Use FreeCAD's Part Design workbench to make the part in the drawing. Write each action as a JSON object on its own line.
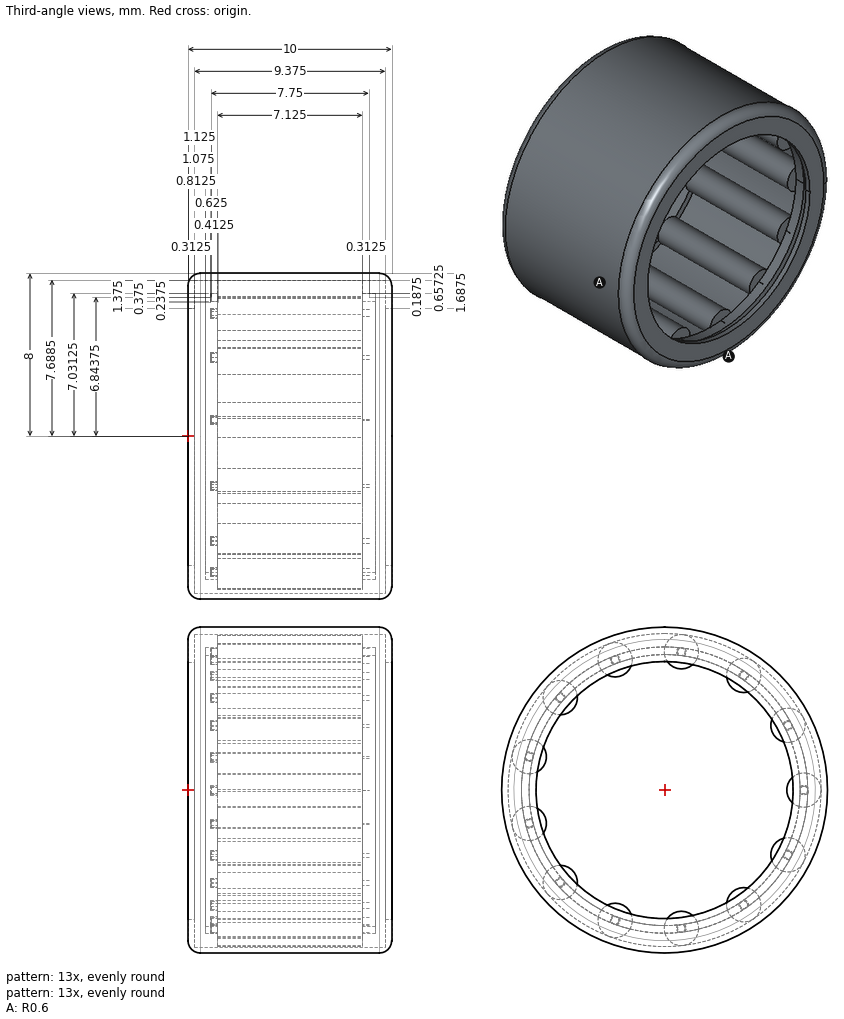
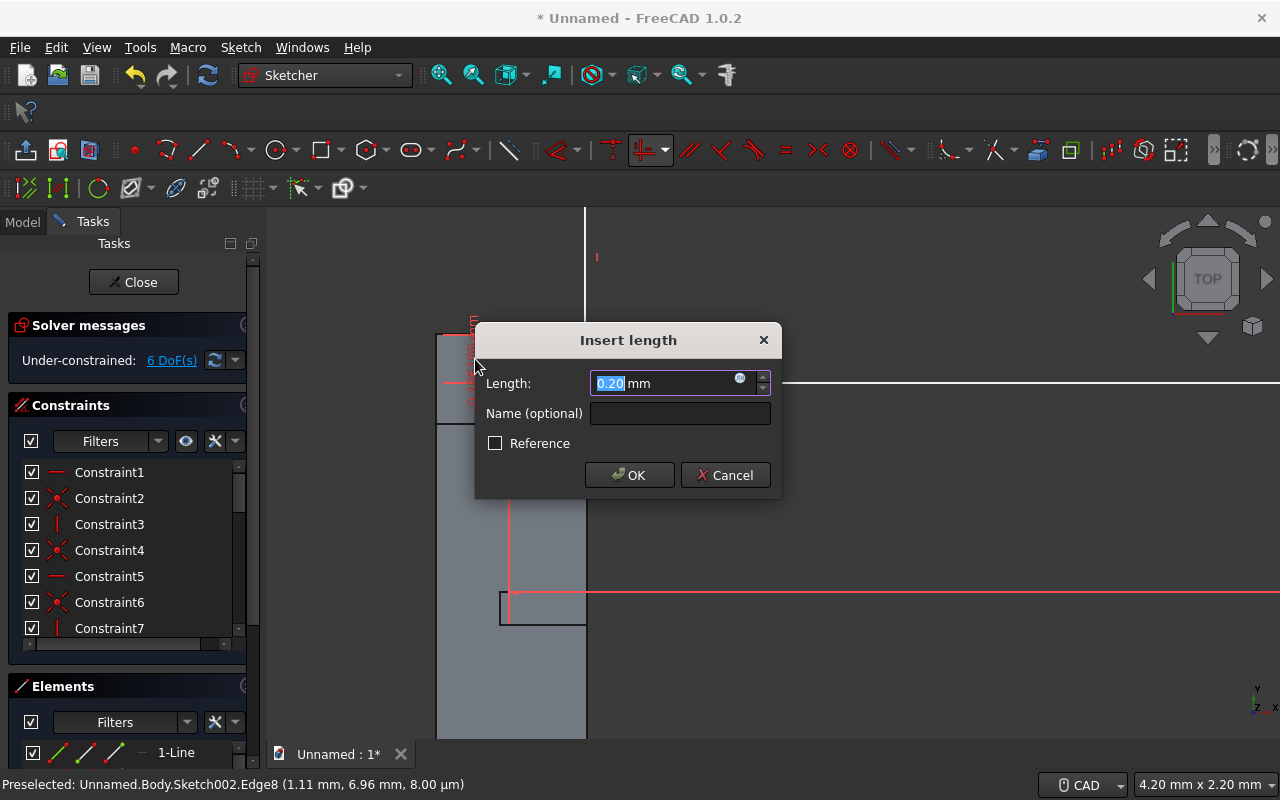
{"action": "type", "text": "0.1875"}
{"action": "key", "text": "Return"}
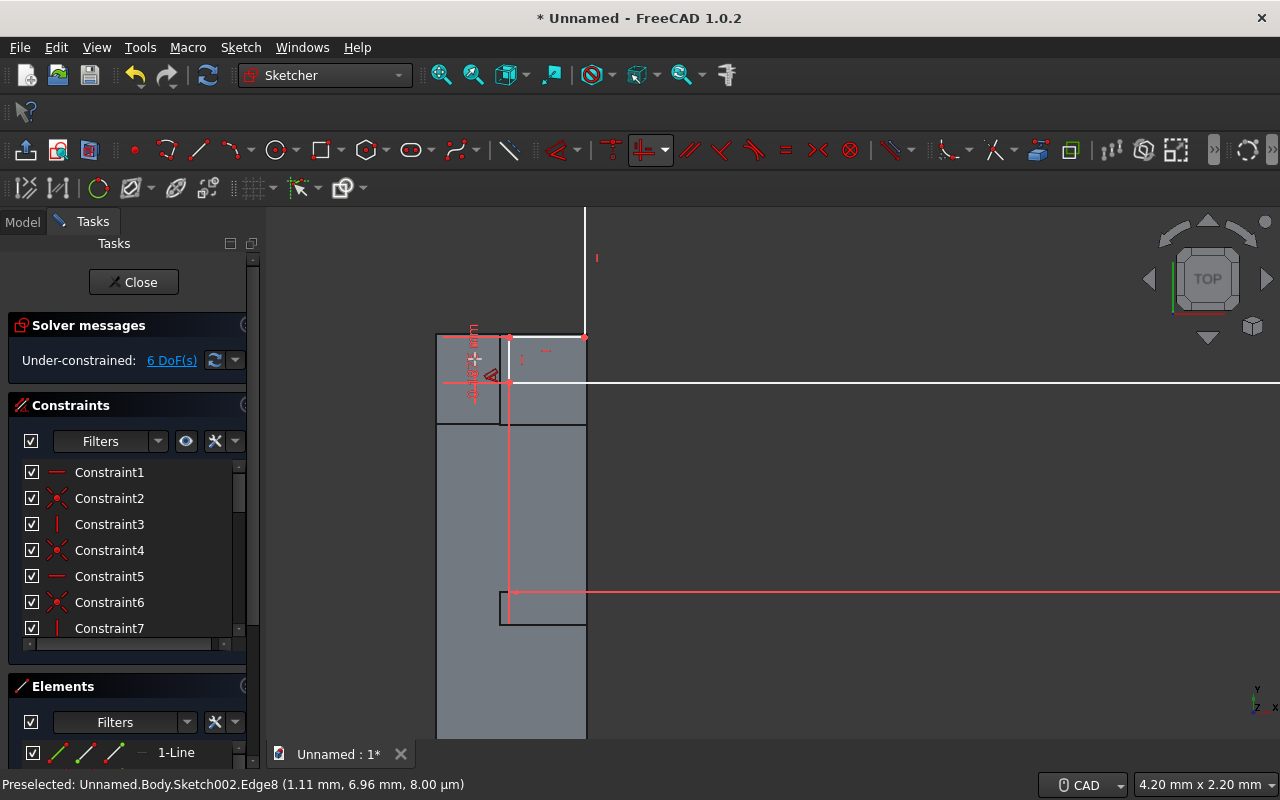
{"action": "scroll", "coordinate": [510, 348], "scroll_direction": "down", "scroll_amount": 9}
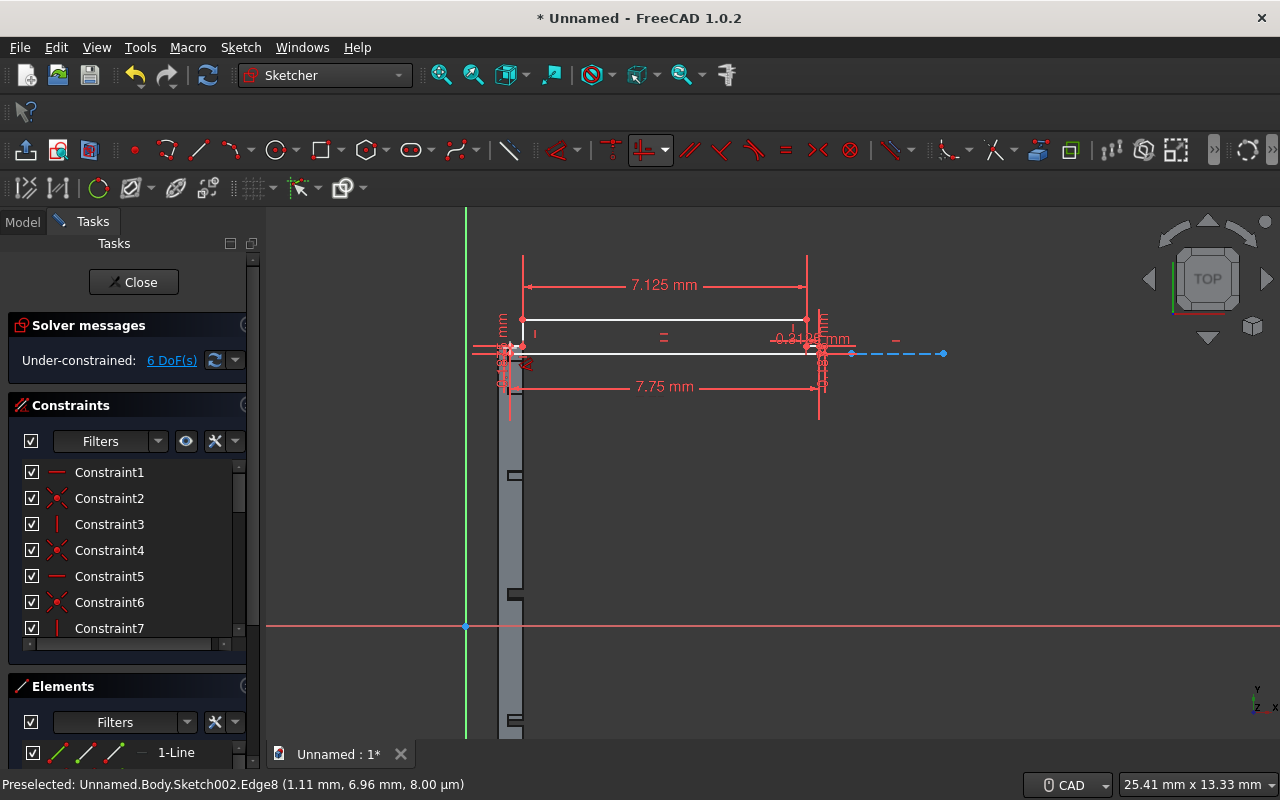
{"action": "scroll", "coordinate": [510, 354], "scroll_direction": "up", "scroll_amount": 3}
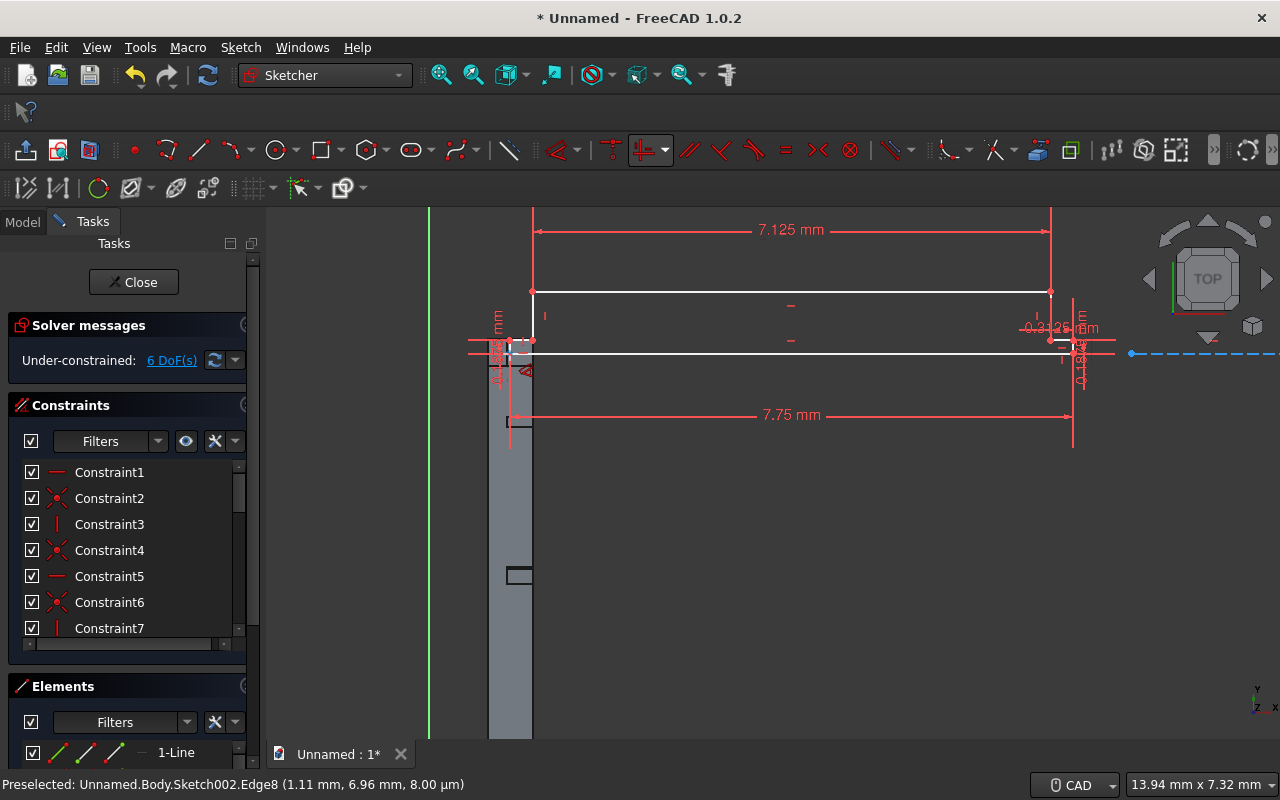
{"action": "left_click", "coordinate": [510, 354]}
{"action": "left_click", "coordinate": [469, 320]}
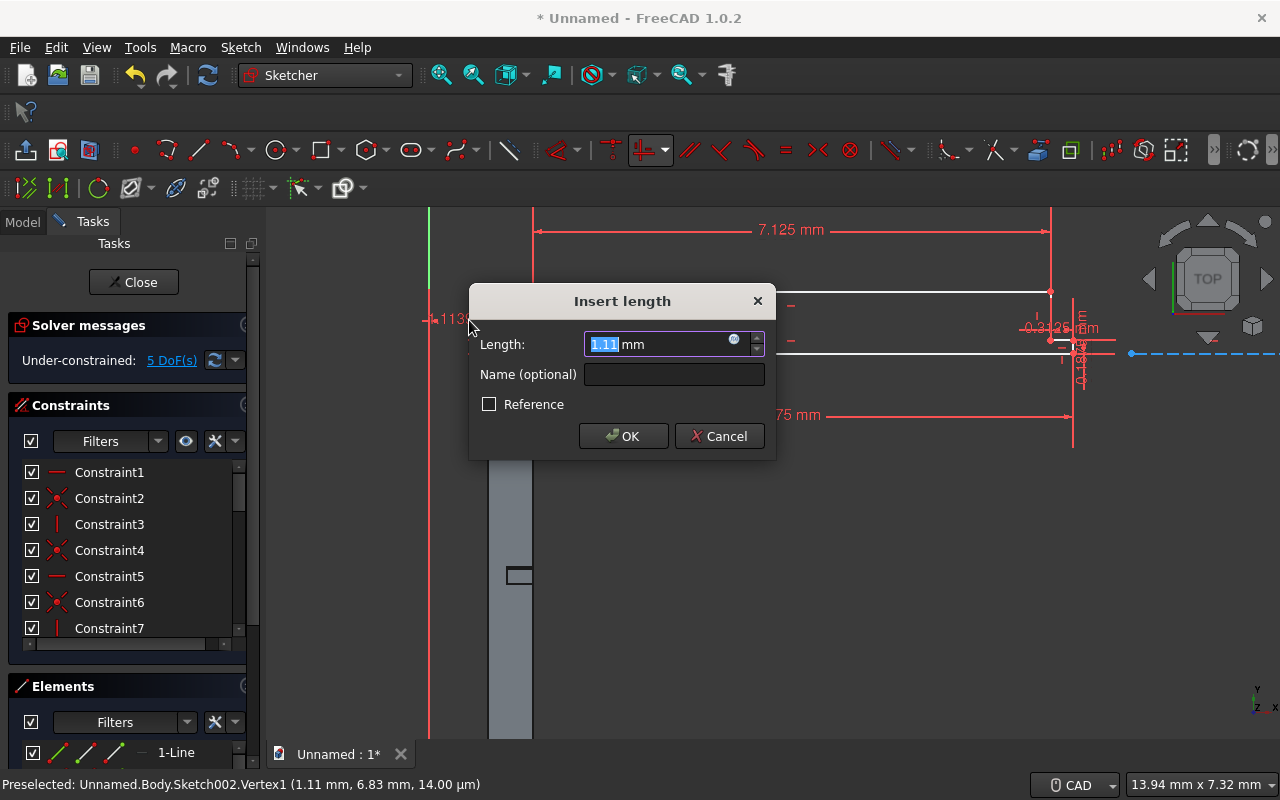
{"action": "type", "text": "1.125"}
{"action": "key", "text": "Return"}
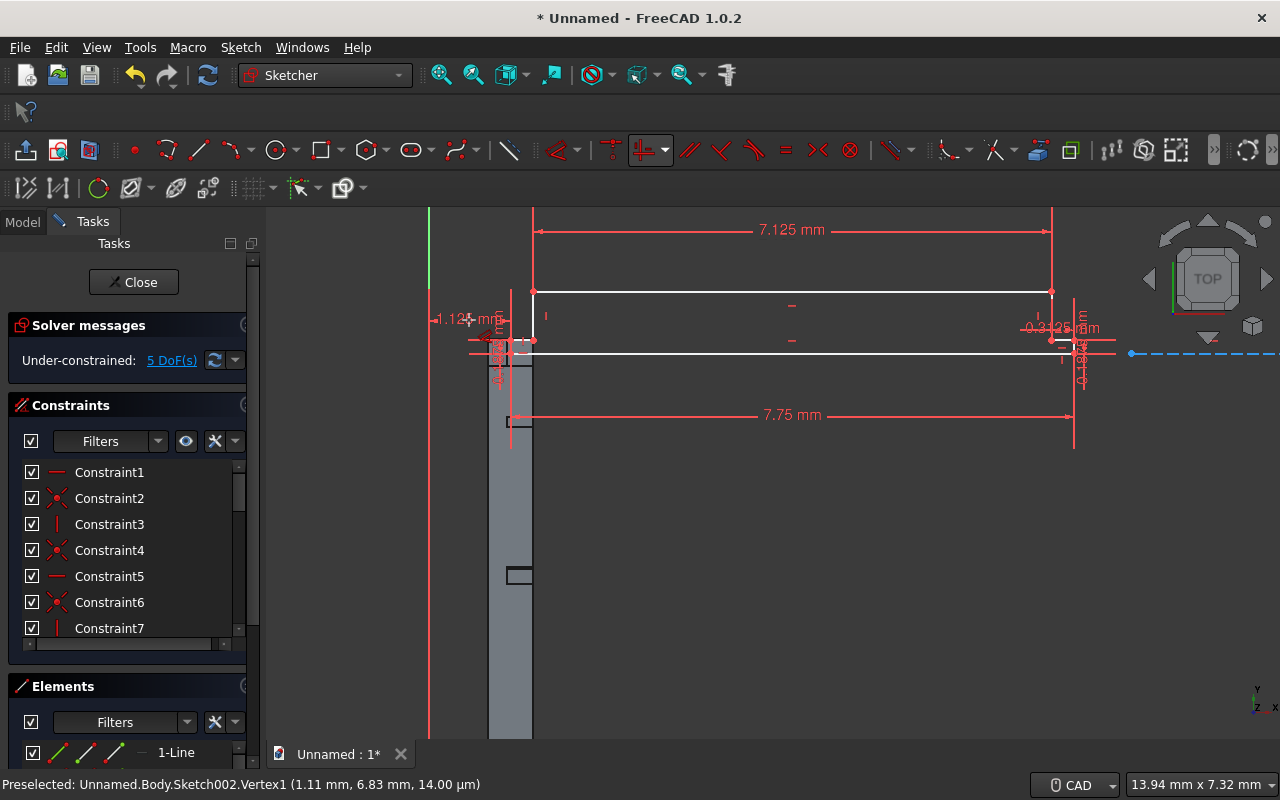
{"action": "left_click", "coordinate": [1052, 326]}
{"action": "left_click", "coordinate": [1086, 305]}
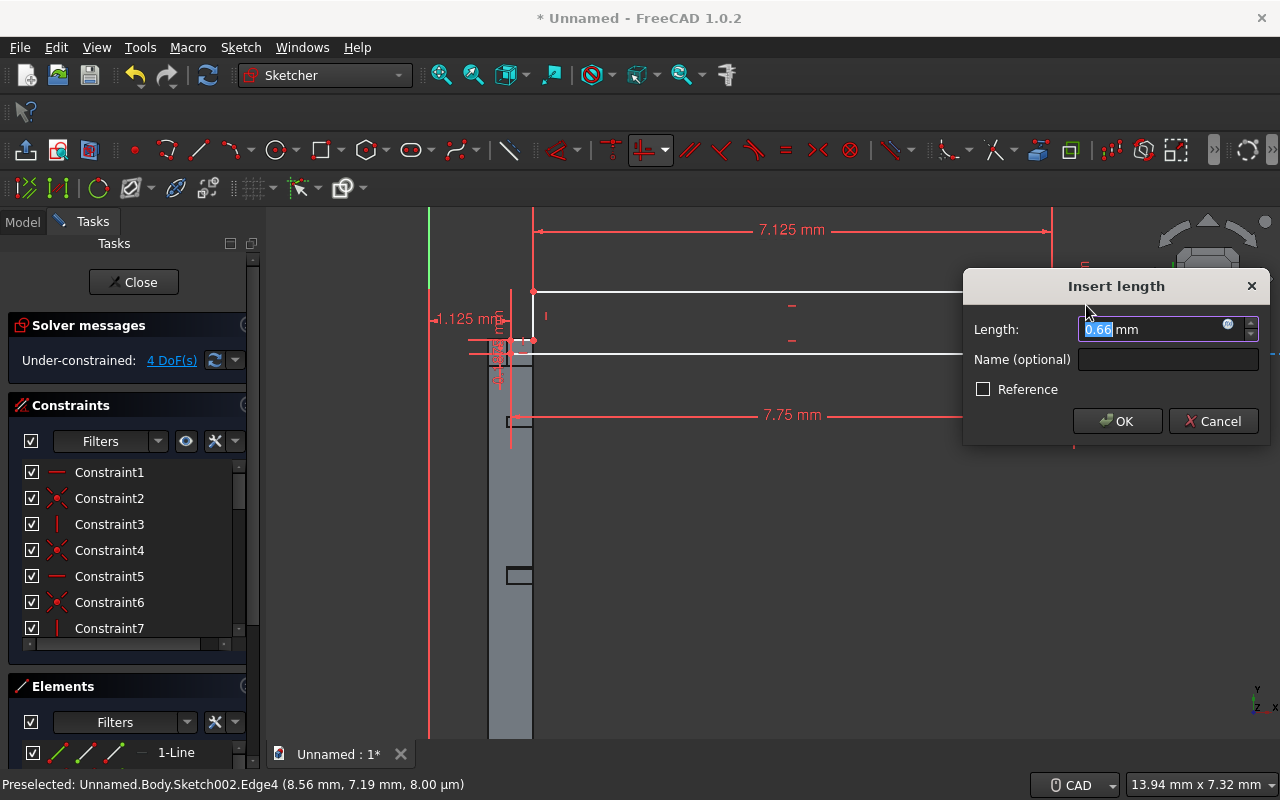
{"action": "type", "text": "0.65725"}
{"action": "key", "text": "Return"}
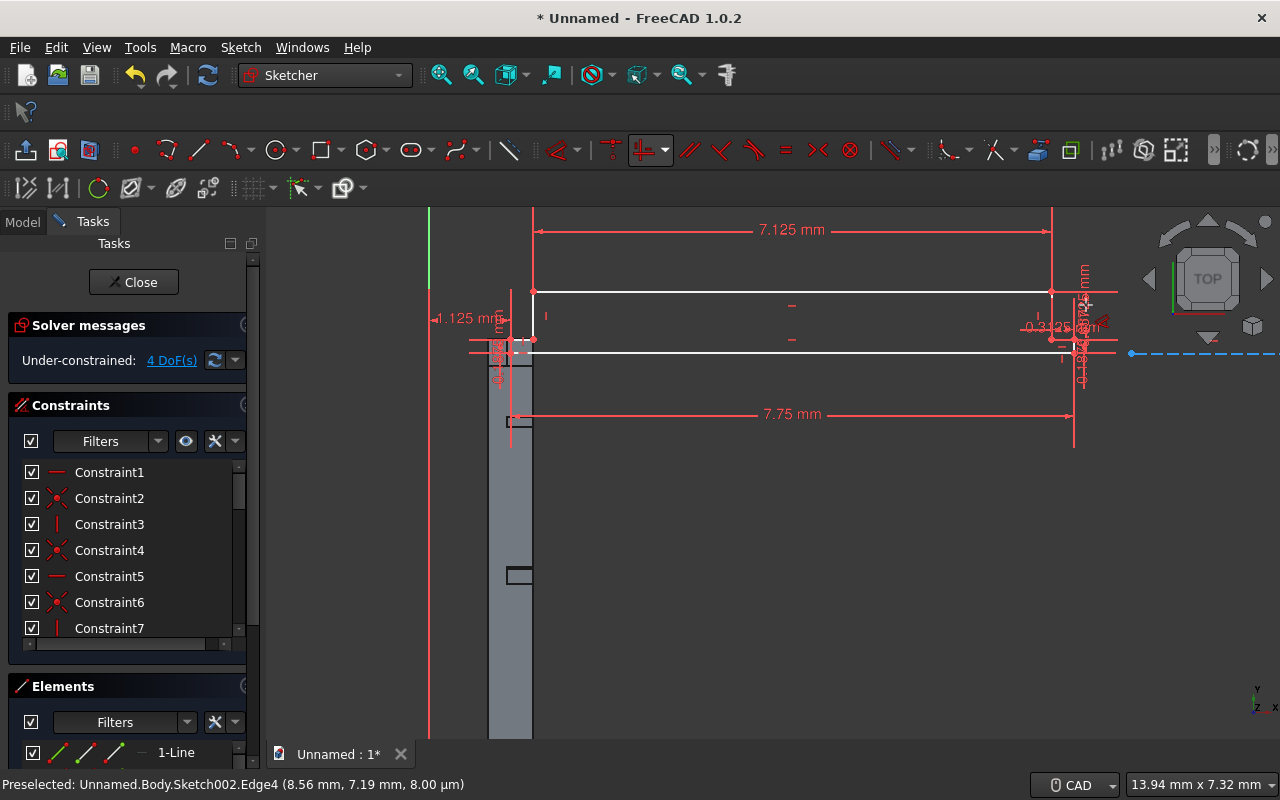
{"action": "left_click", "coordinate": [1052, 292]}
{"action": "left_click", "coordinate": [395, 501]}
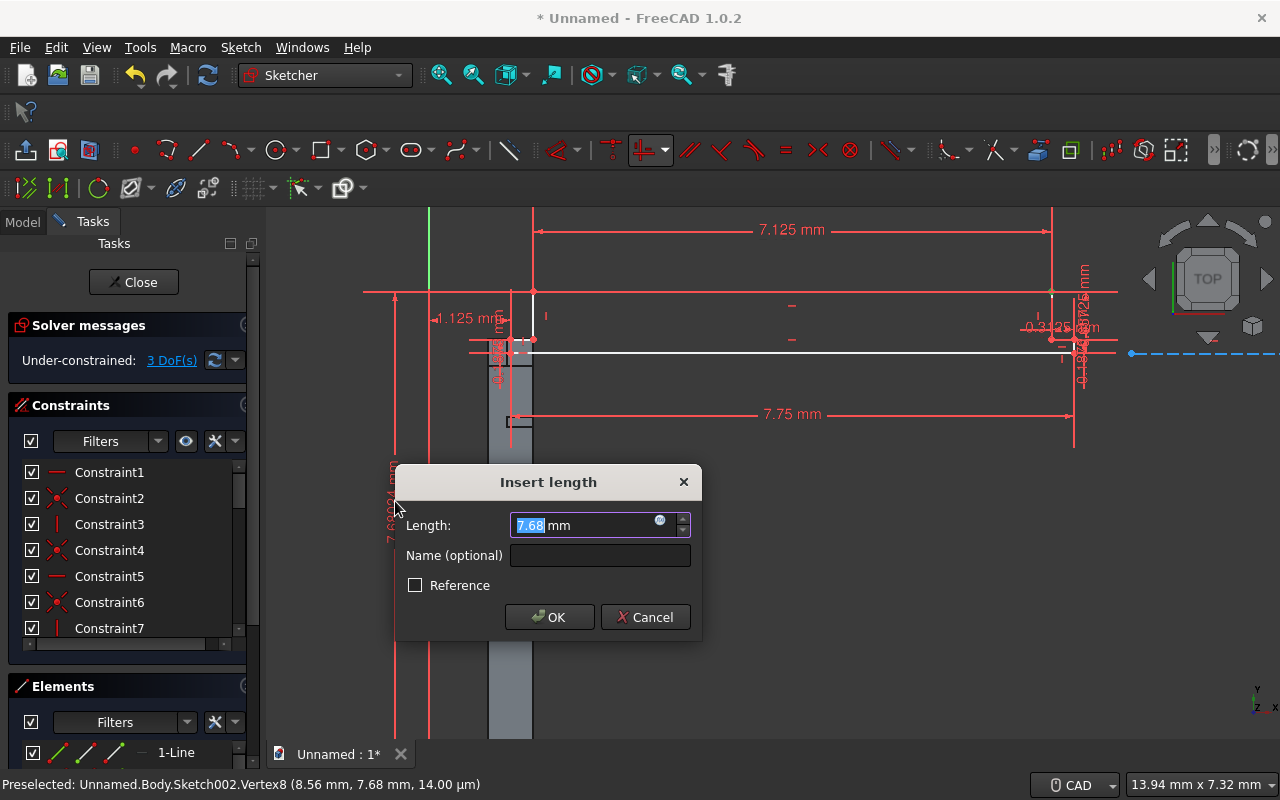
{"action": "type", "text": "7.6885"}
{"action": "key", "text": "Return"}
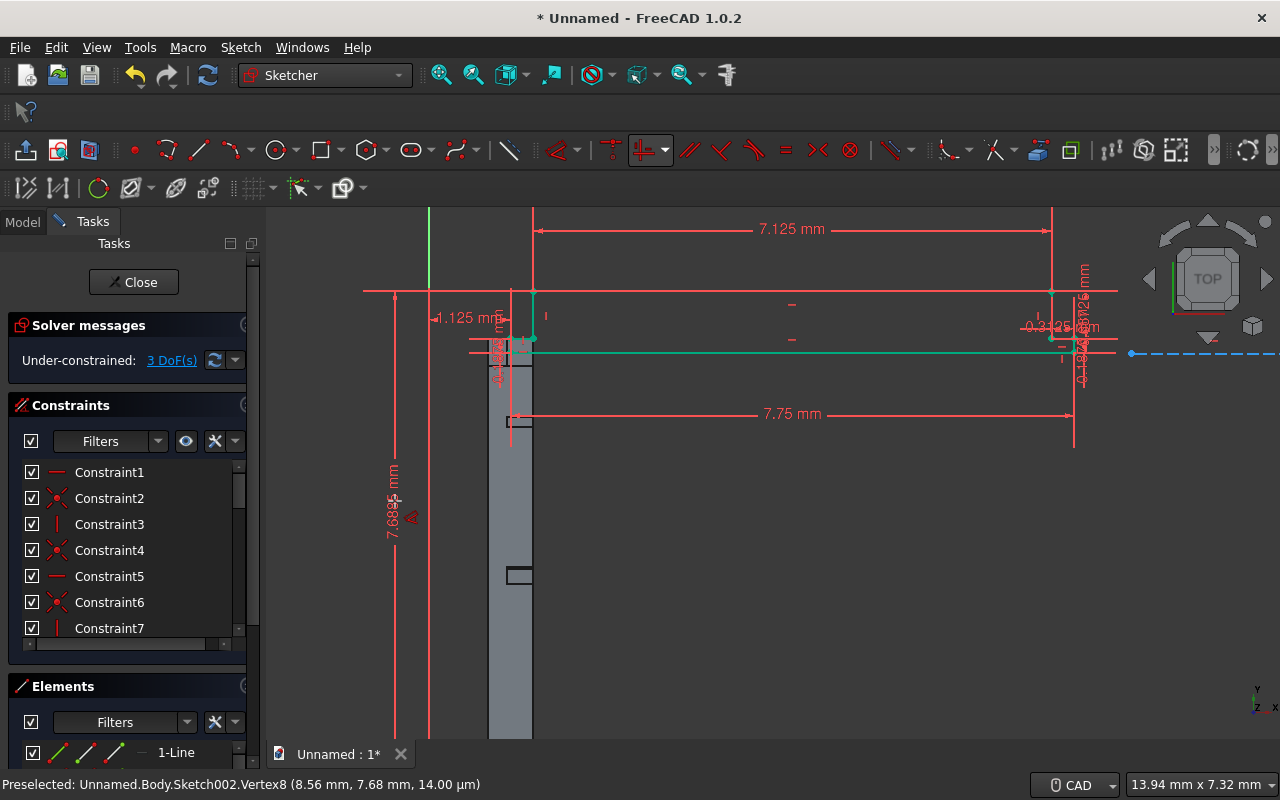
{"action": "scroll", "coordinate": [510, 354], "scroll_direction": "down", "scroll_amount": 3}